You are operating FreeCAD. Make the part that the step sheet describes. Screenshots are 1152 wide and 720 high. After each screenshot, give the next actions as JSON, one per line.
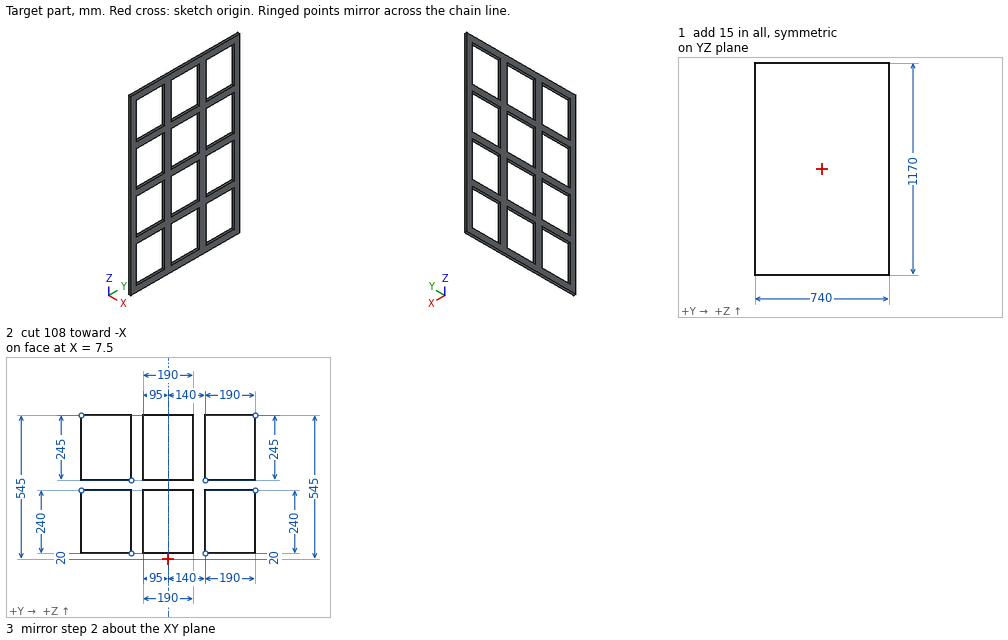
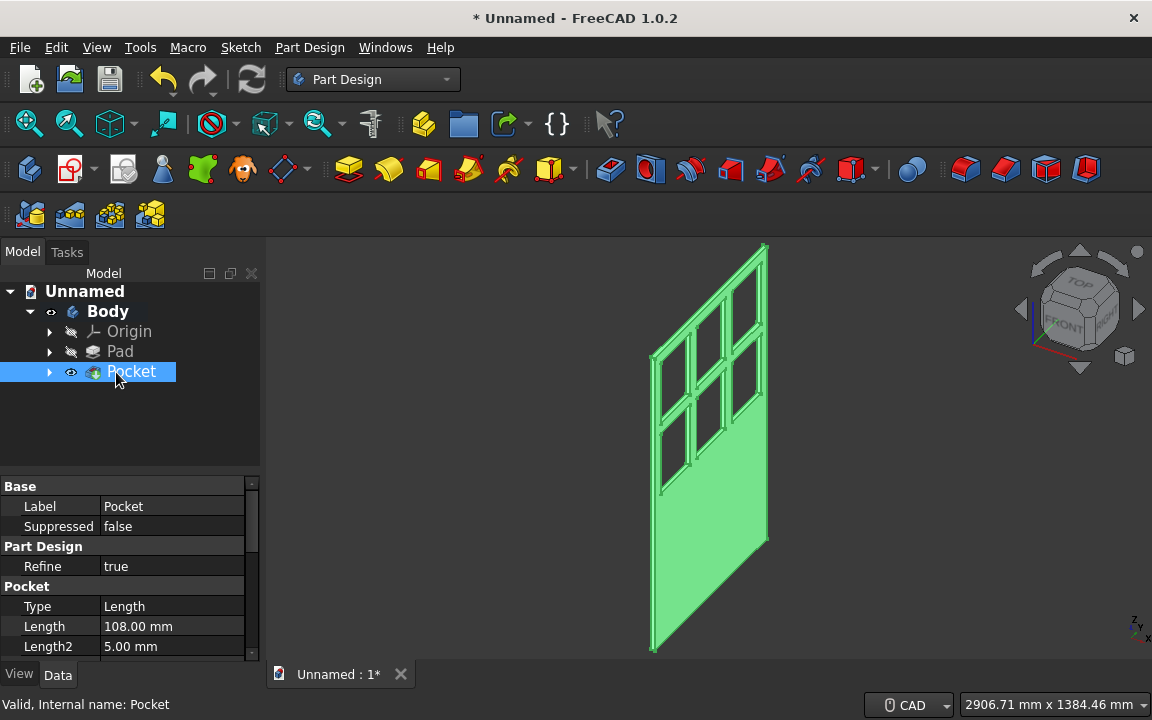
{"action": "left_click", "coordinate": [30, 214]}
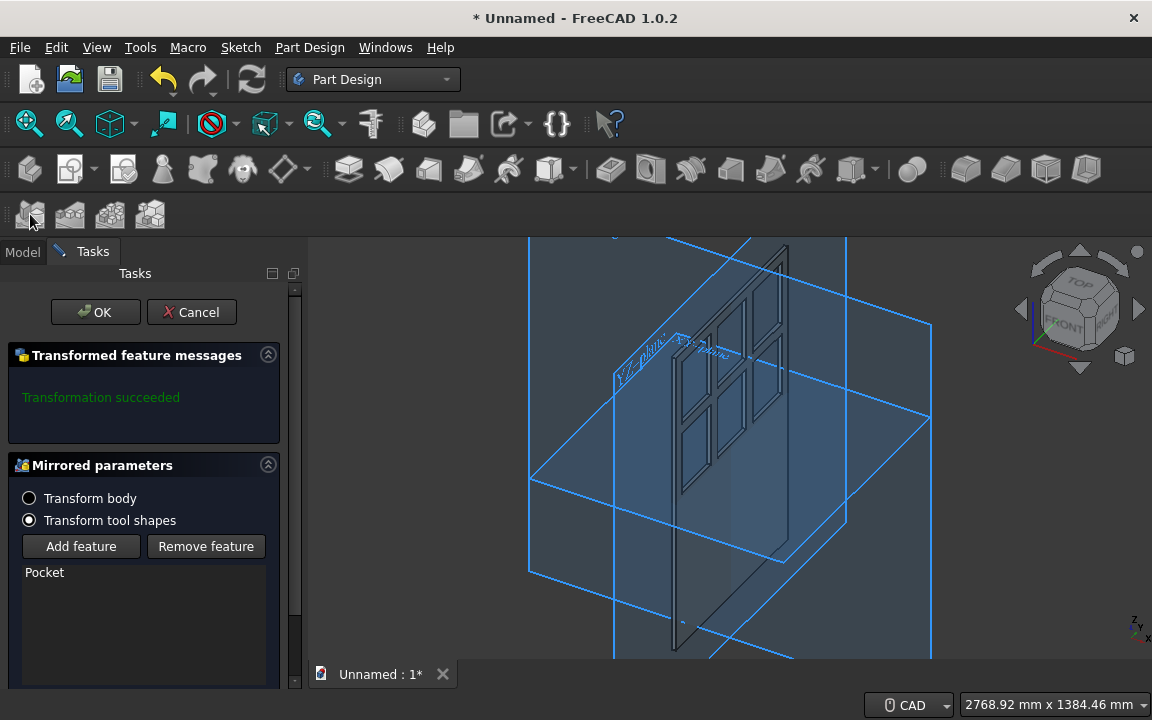
{"action": "scroll", "coordinate": [295, 486], "scroll_direction": "down", "scroll_amount": 2}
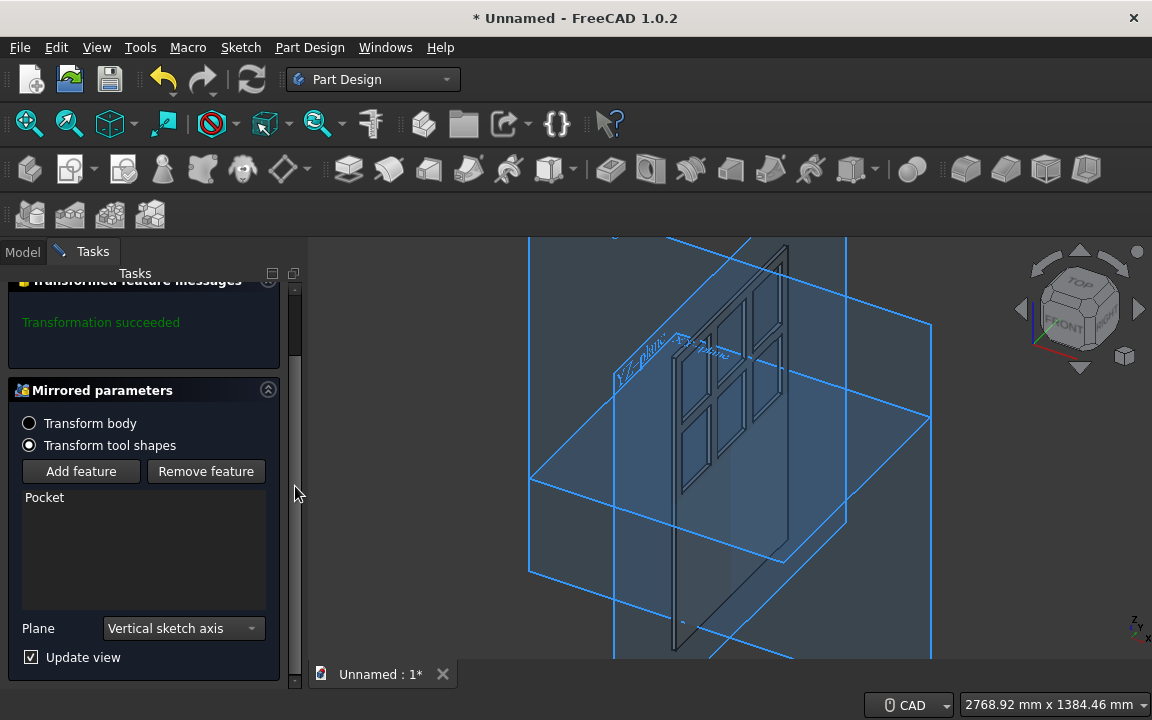
{"action": "left_click", "coordinate": [184, 628]}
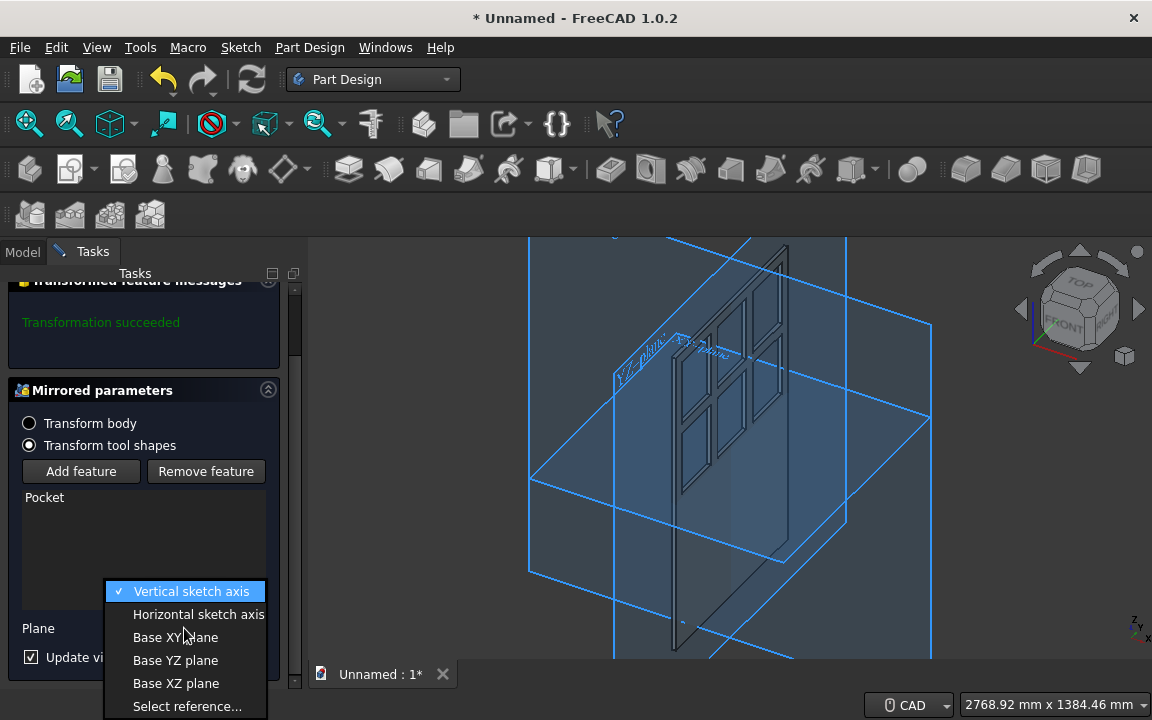
{"action": "left_click", "coordinate": [184, 638]}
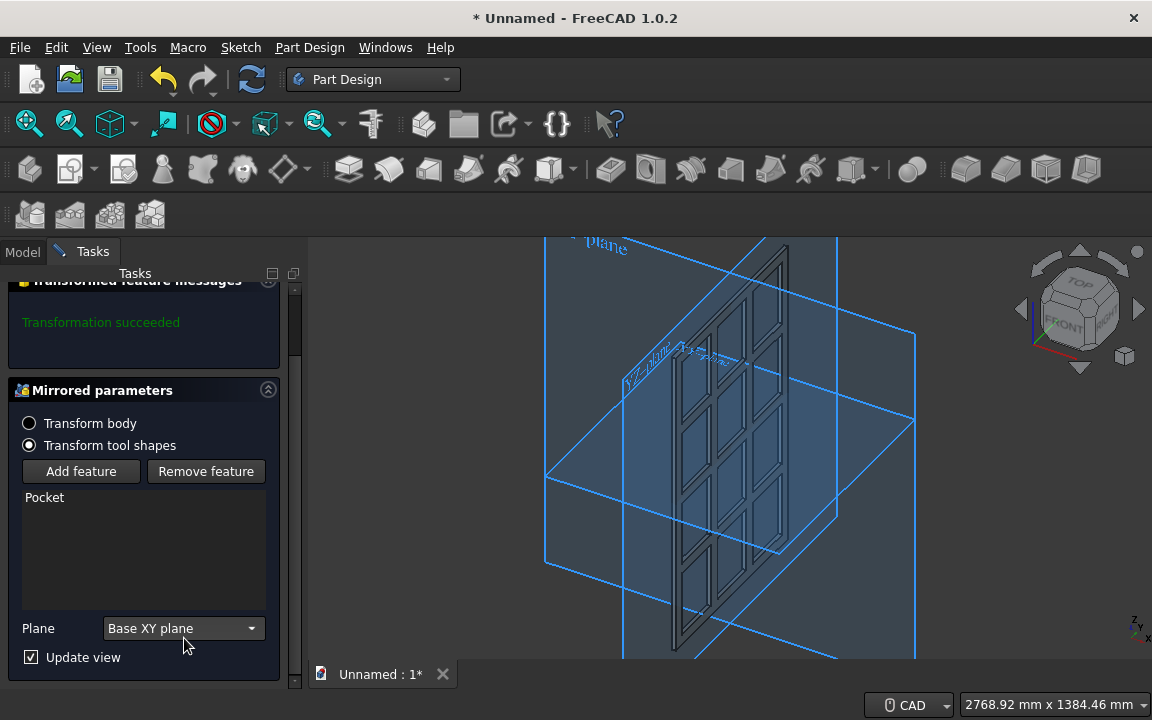
{"action": "scroll", "coordinate": [295, 486], "scroll_direction": "up", "scroll_amount": 2}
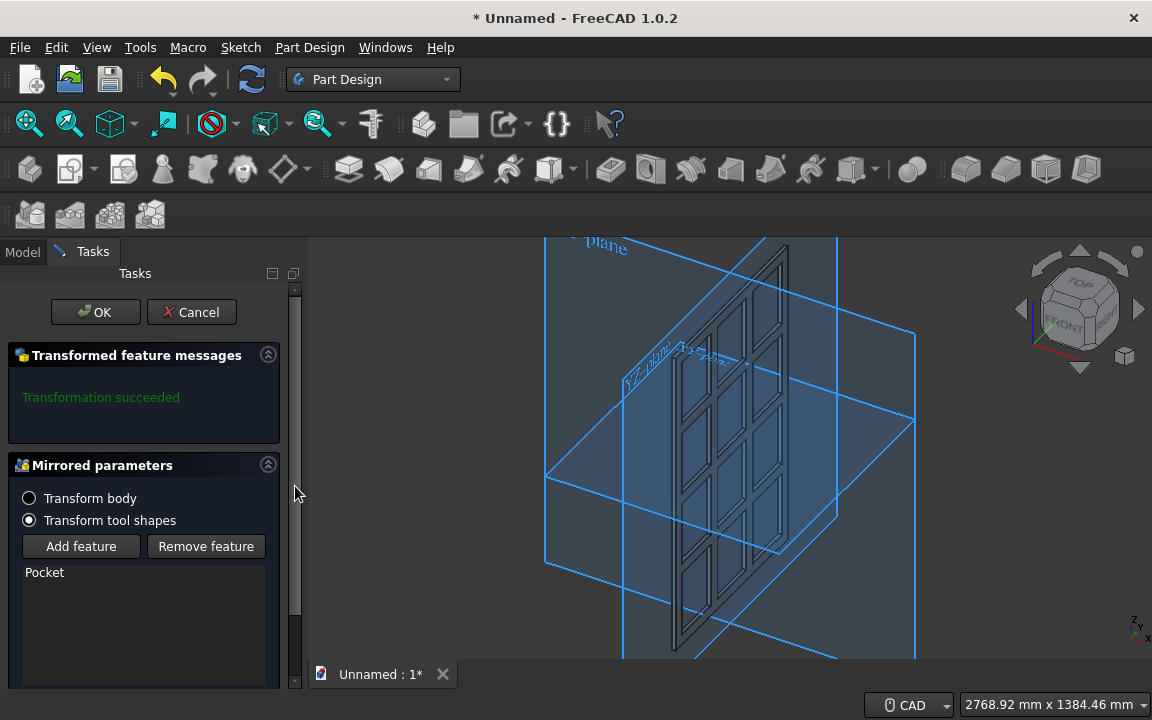
{"action": "left_click", "coordinate": [96, 312]}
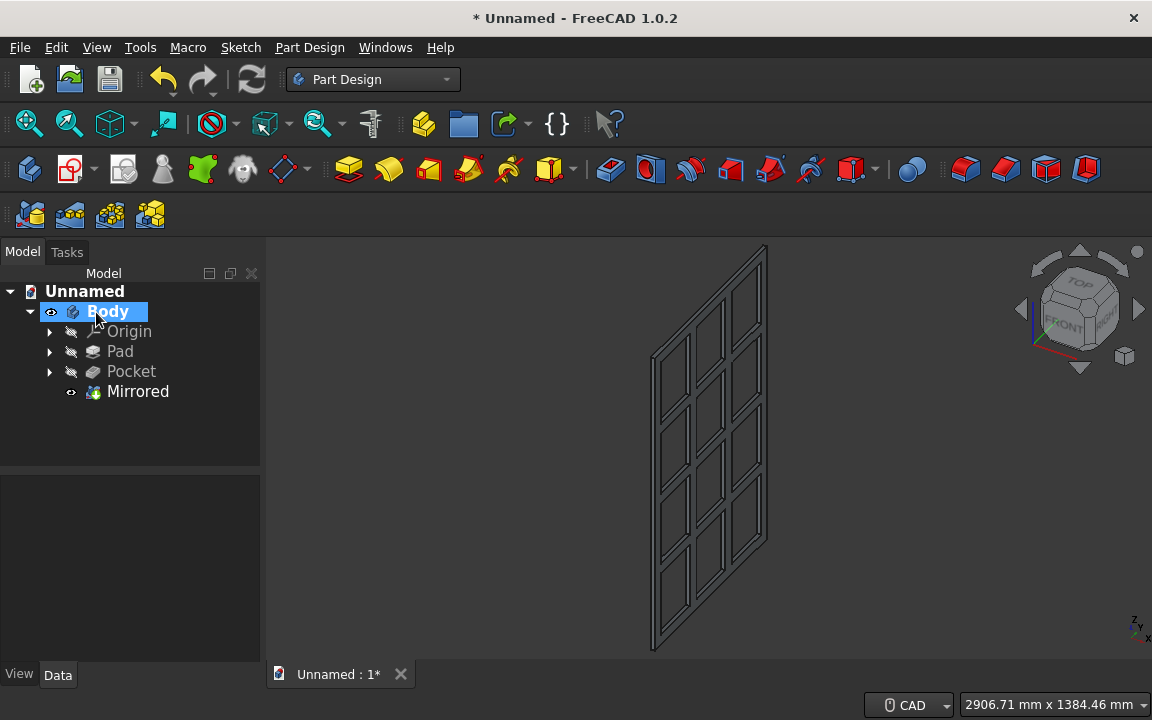
{"action": "key", "text": "0"}